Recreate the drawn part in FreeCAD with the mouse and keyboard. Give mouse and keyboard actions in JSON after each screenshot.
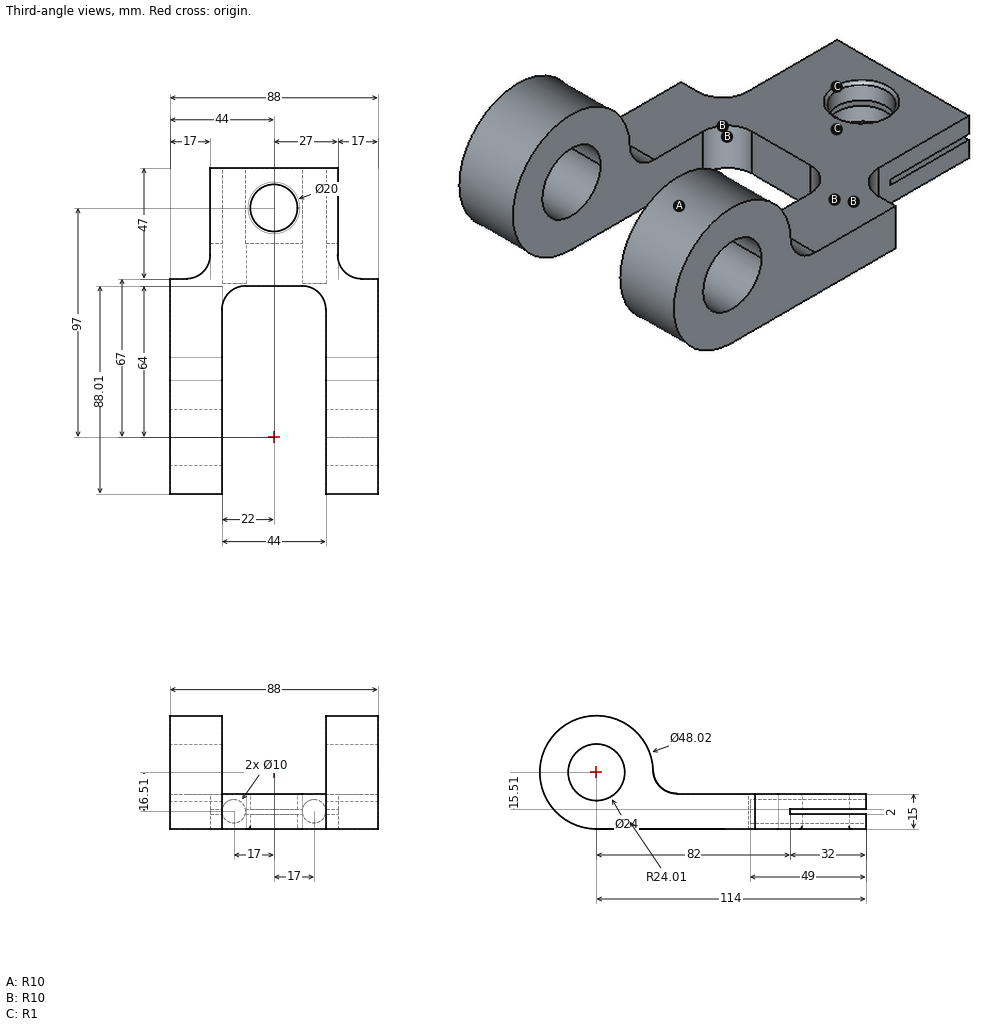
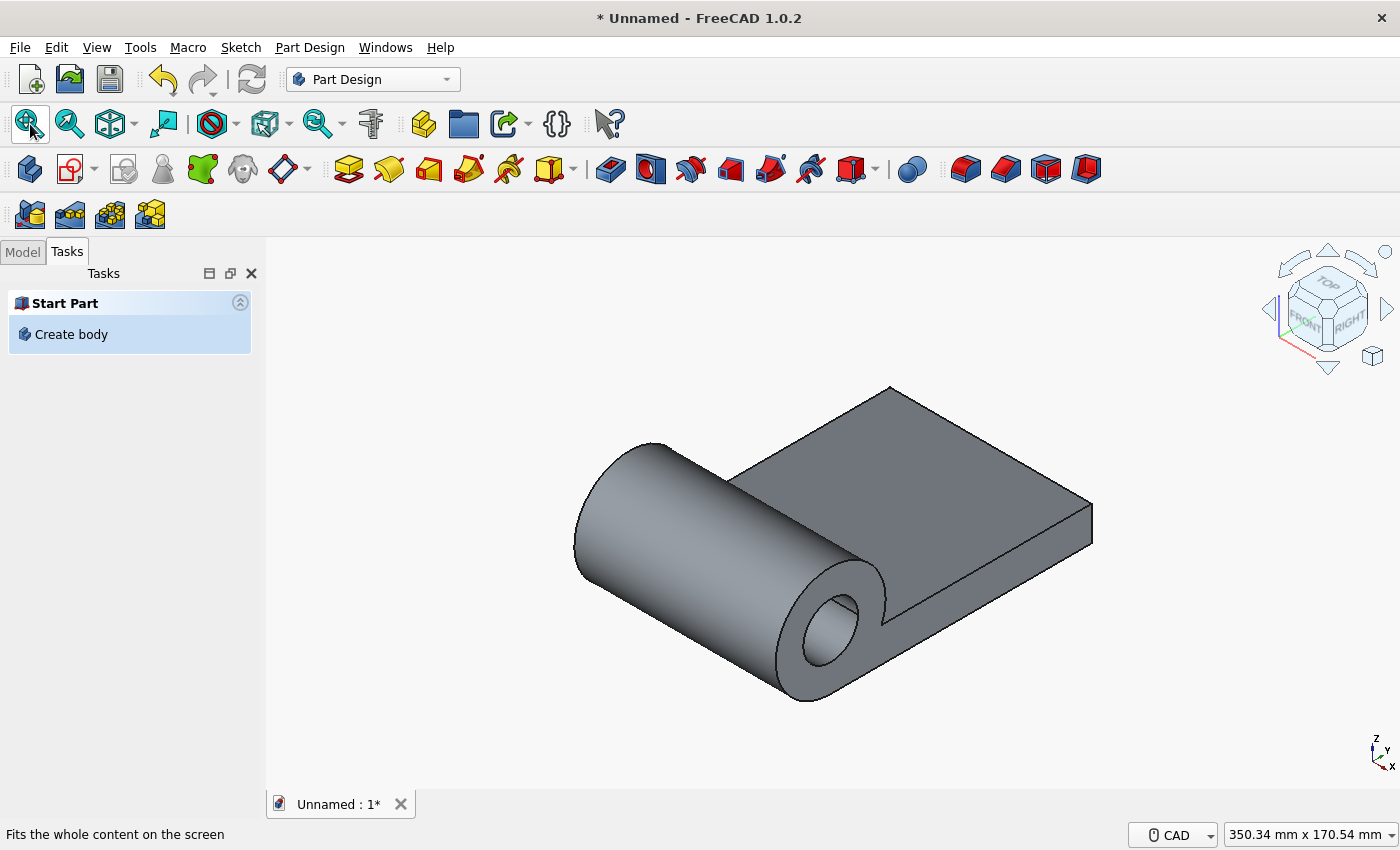
{"action": "key", "text": "2"}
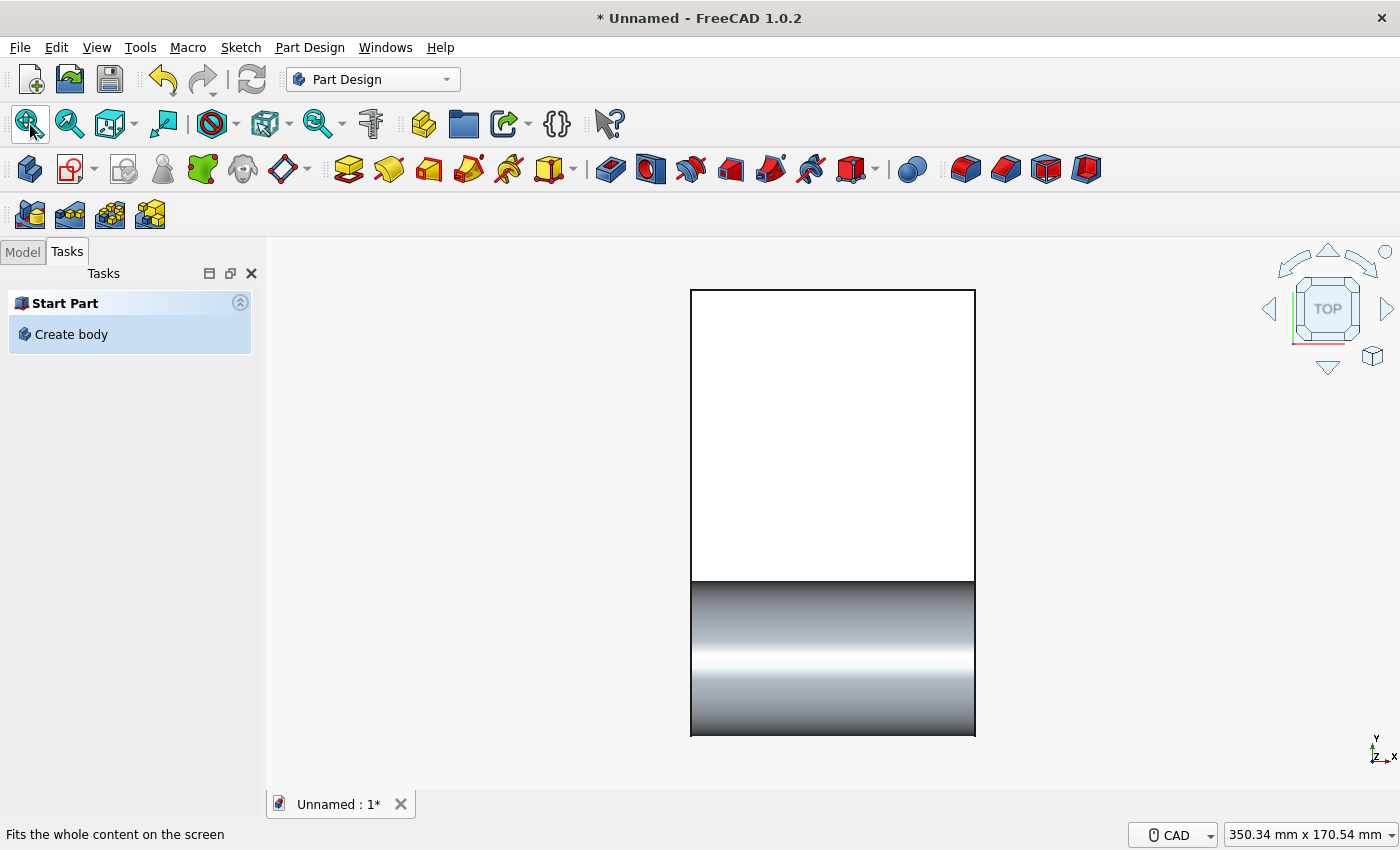
{"action": "key", "text": "1"}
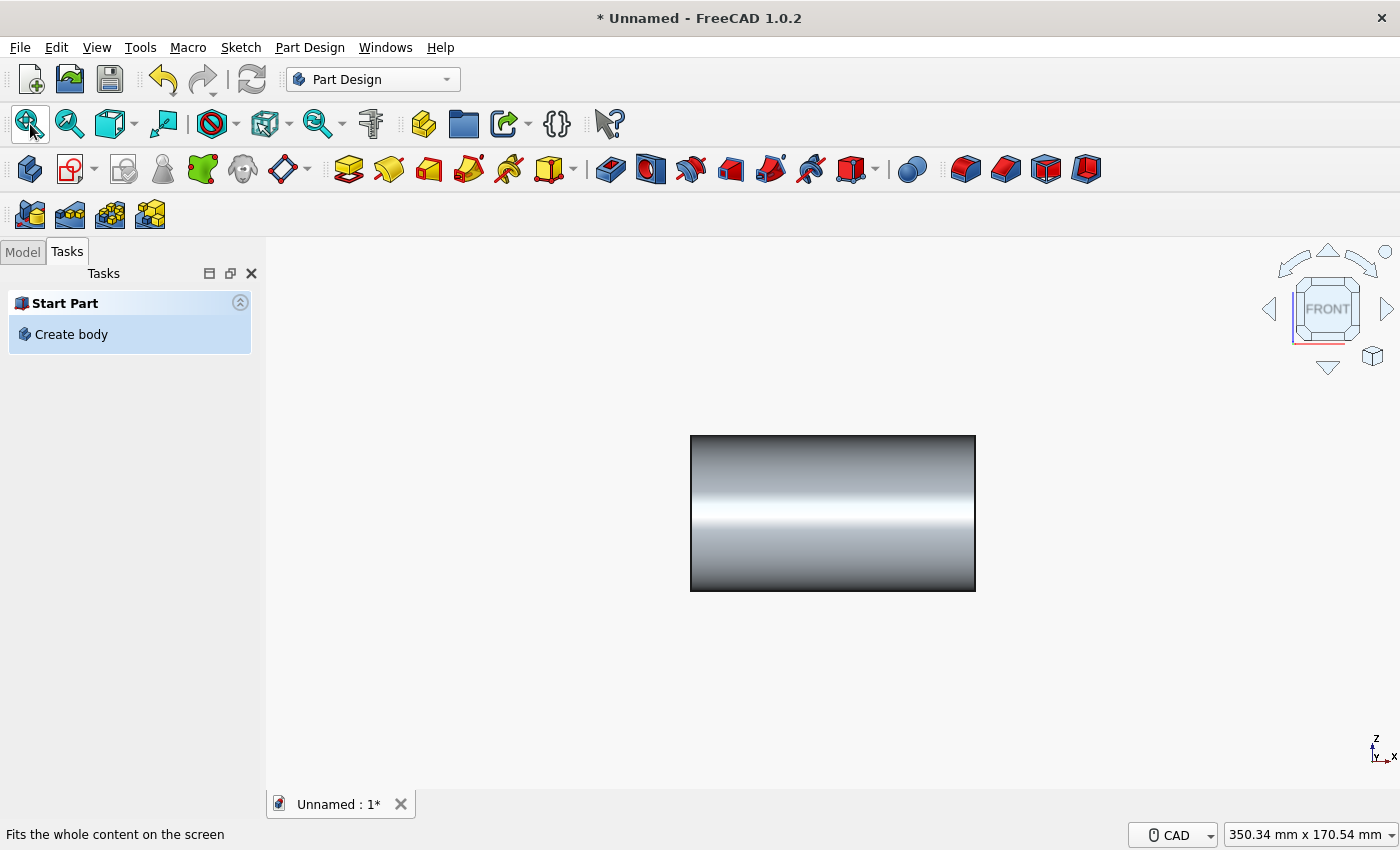
{"action": "left_click", "coordinate": [30, 124]}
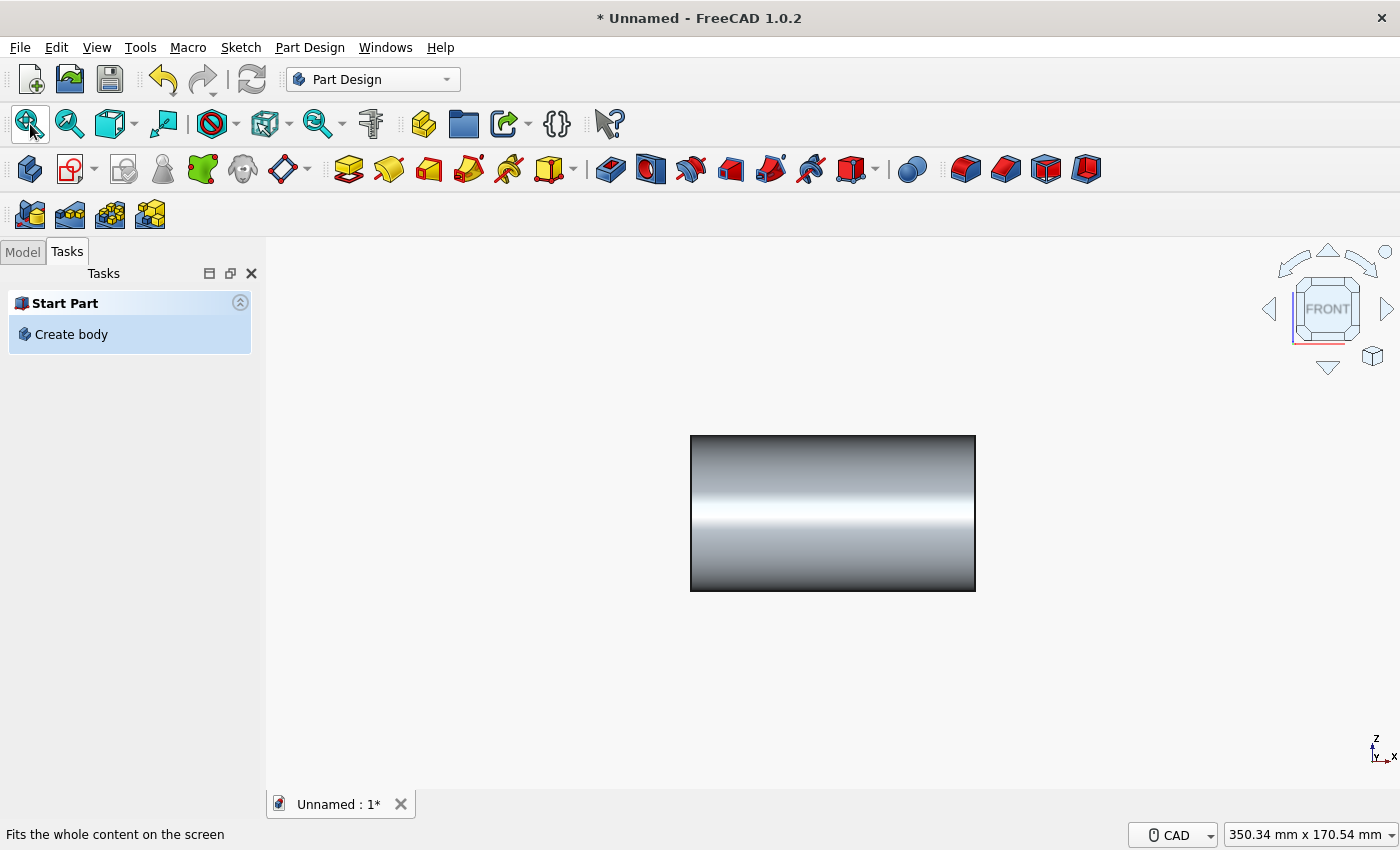
{"action": "key", "text": "3"}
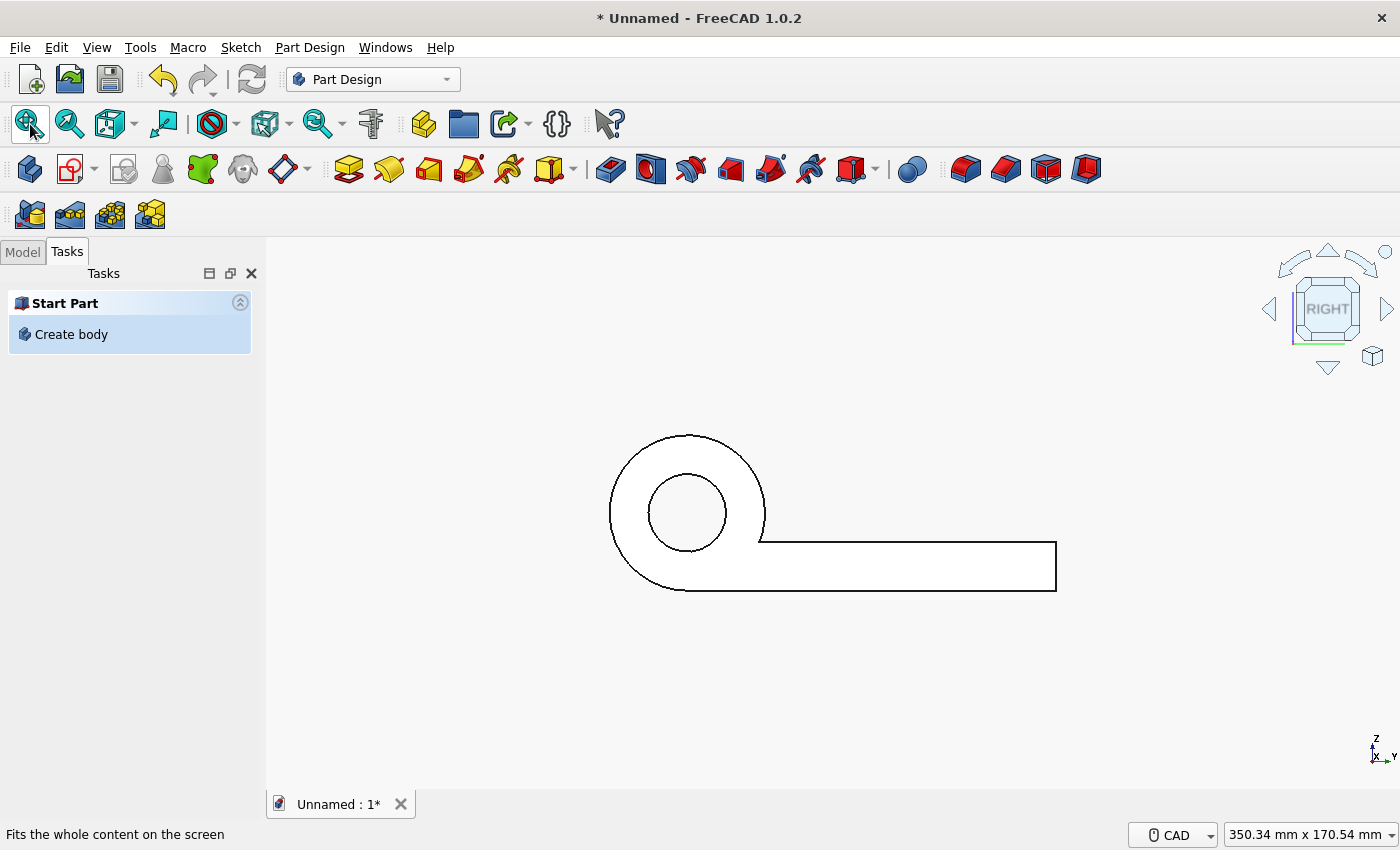
{"action": "left_click", "coordinate": [30, 124]}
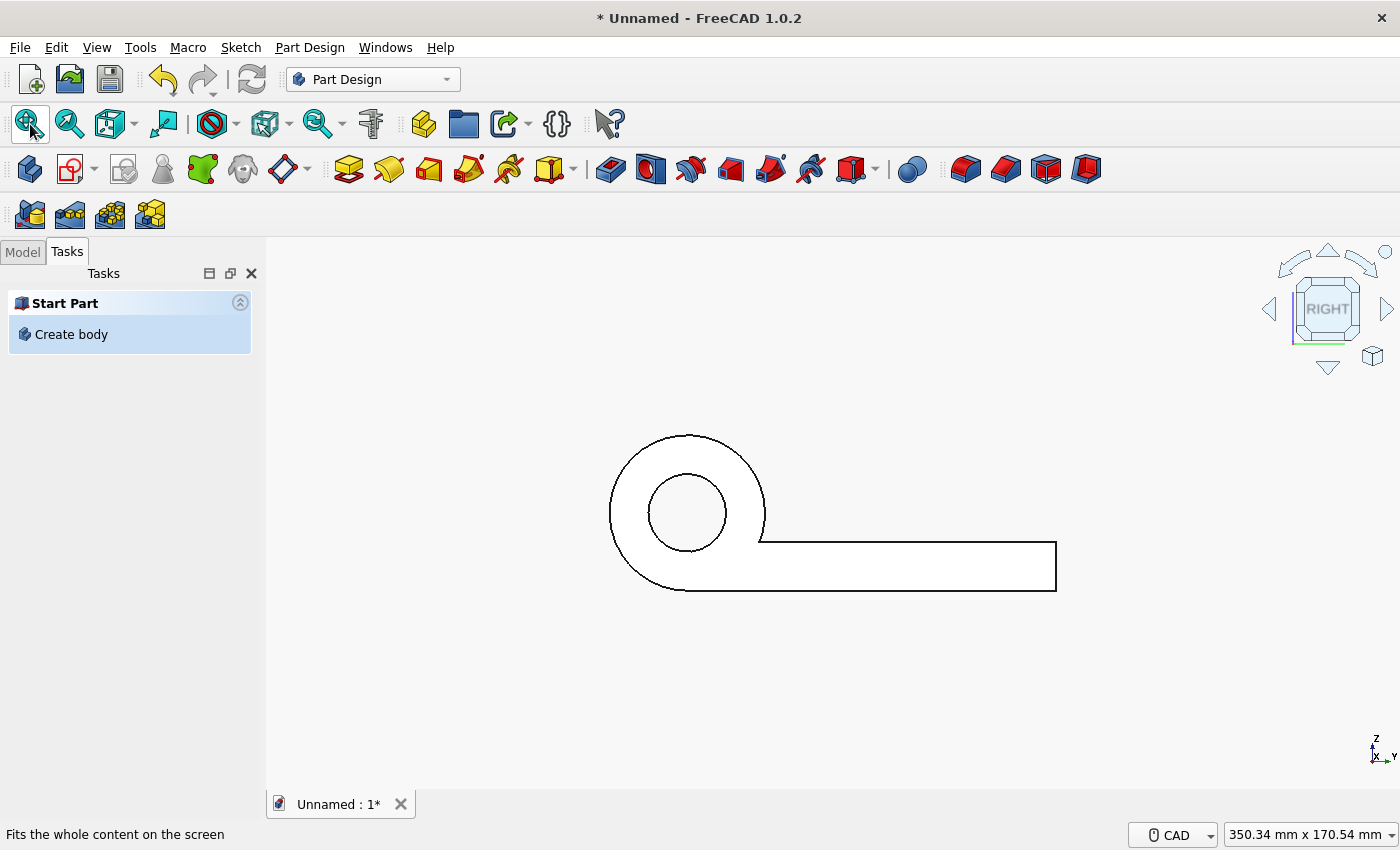
{"action": "key", "text": "5"}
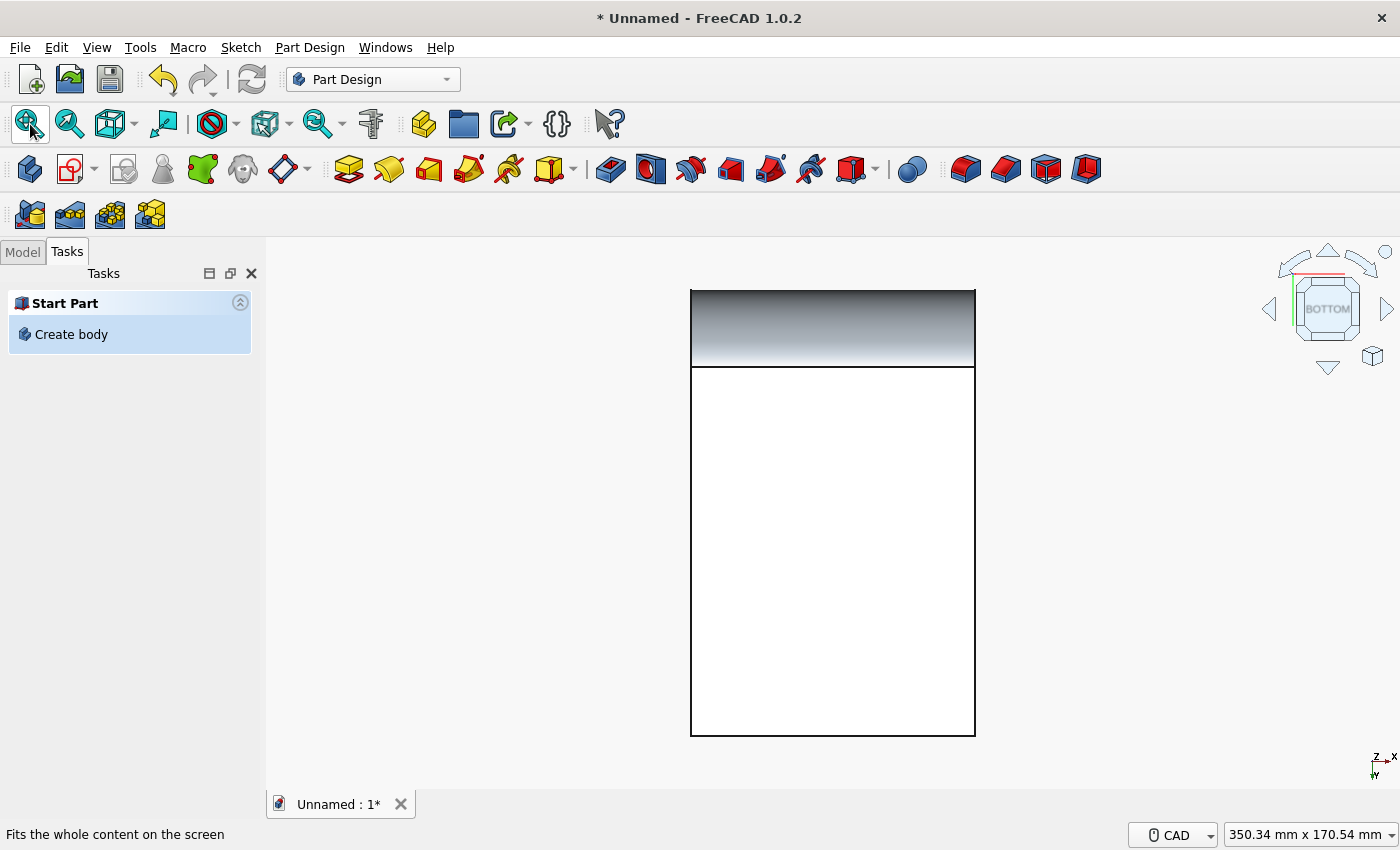
{"action": "key", "text": "4"}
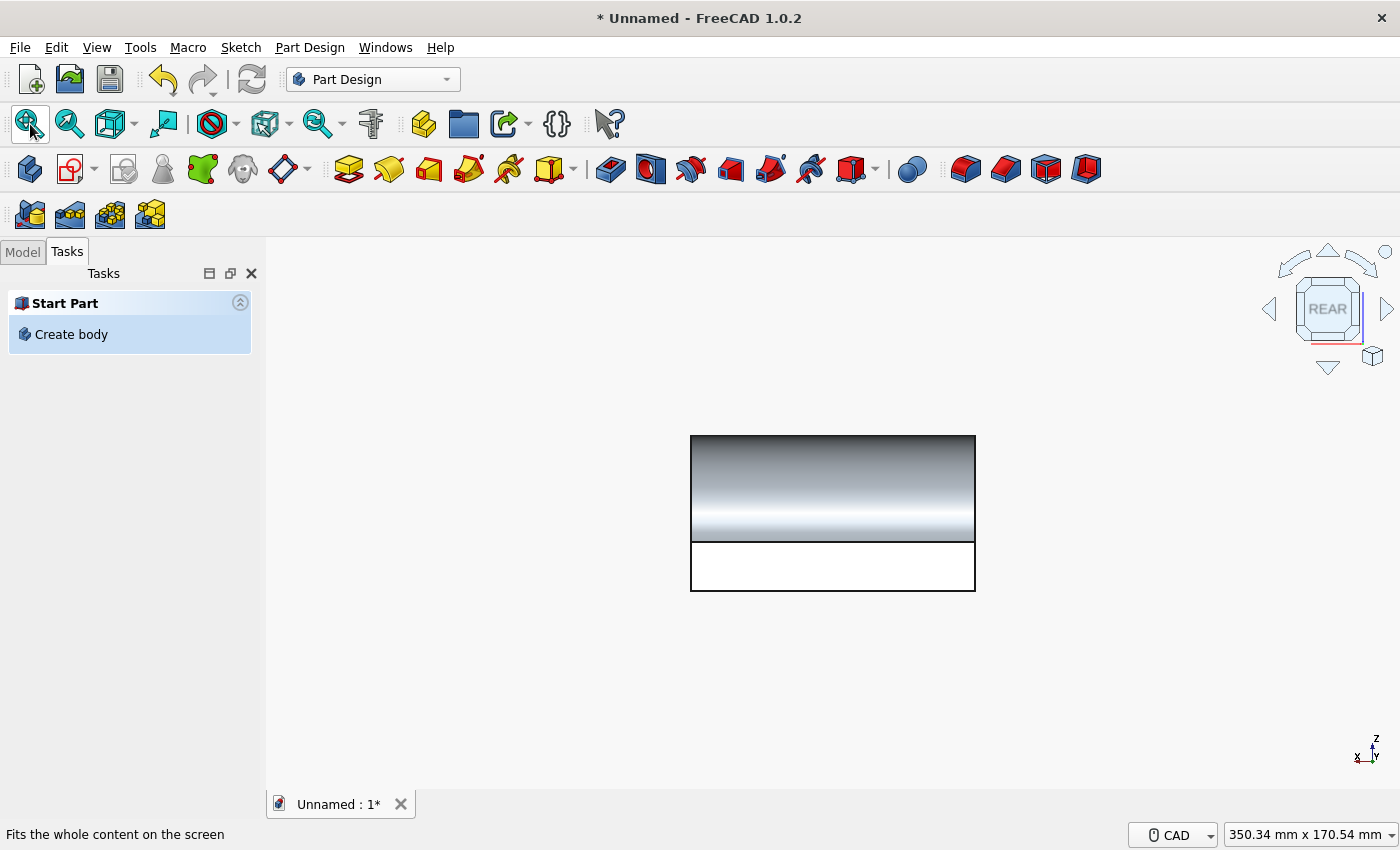
{"action": "left_click", "coordinate": [30, 124]}